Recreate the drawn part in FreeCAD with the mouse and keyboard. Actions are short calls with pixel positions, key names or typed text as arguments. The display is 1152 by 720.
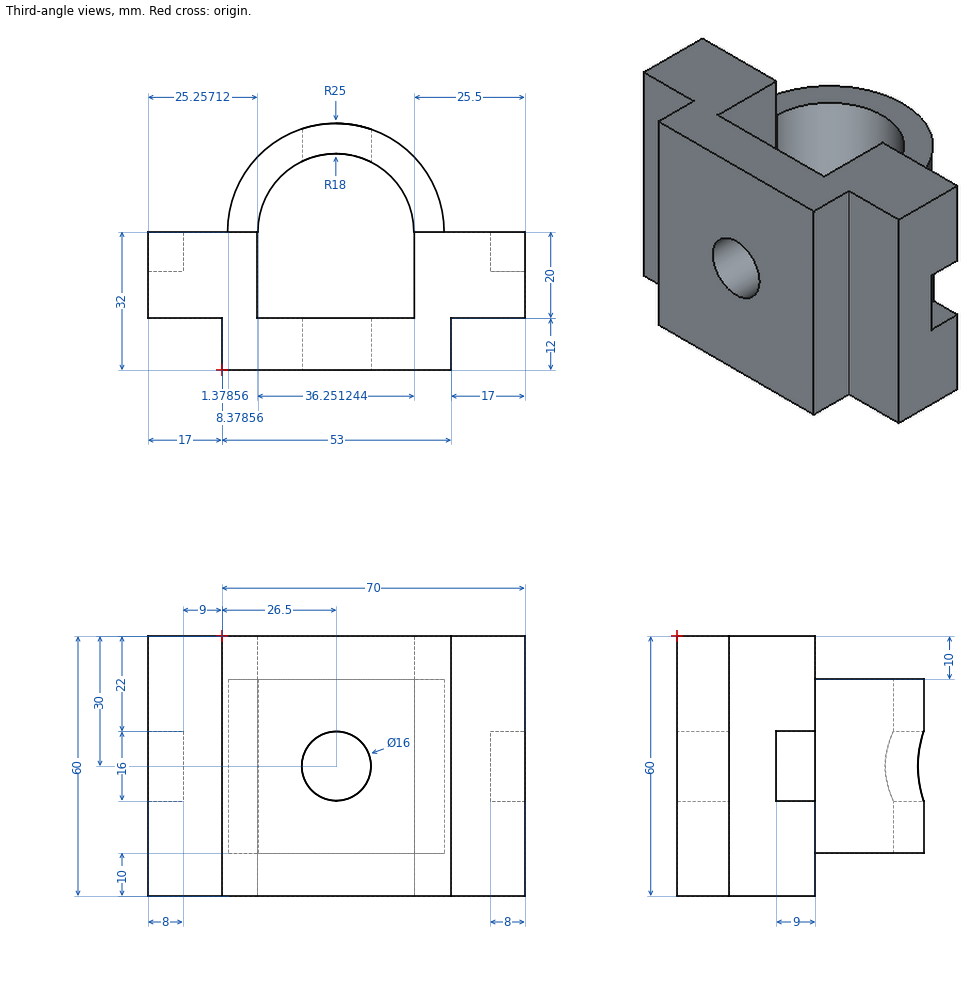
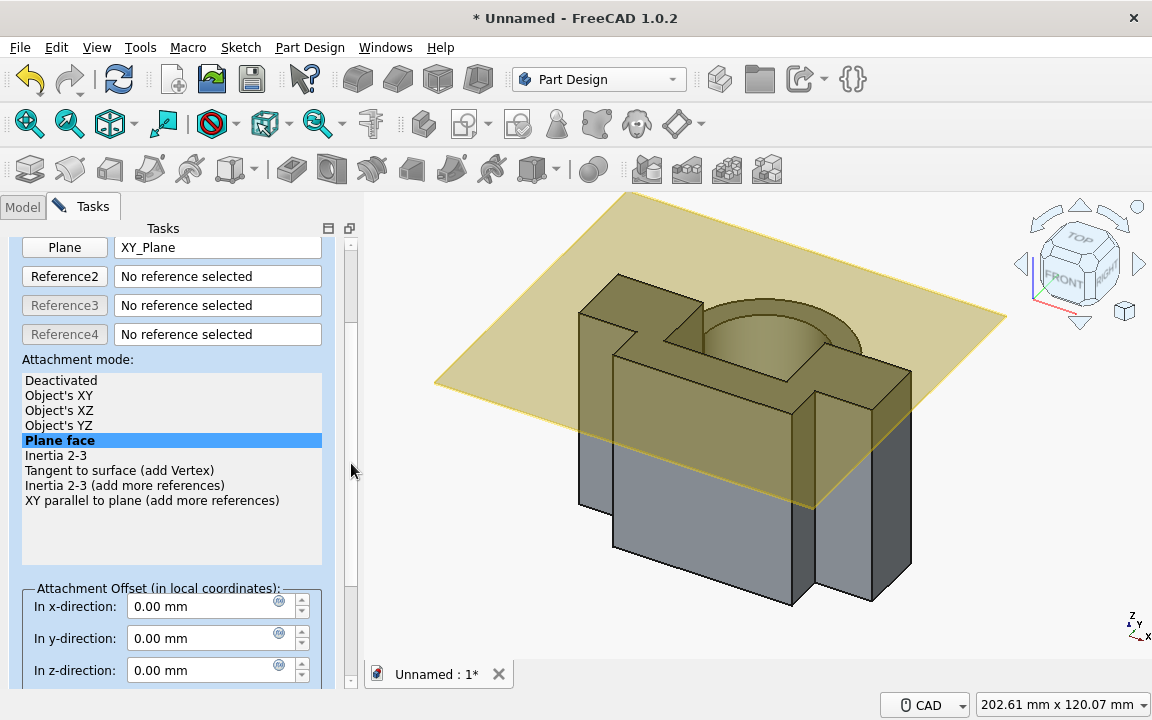
triple_click(210, 610)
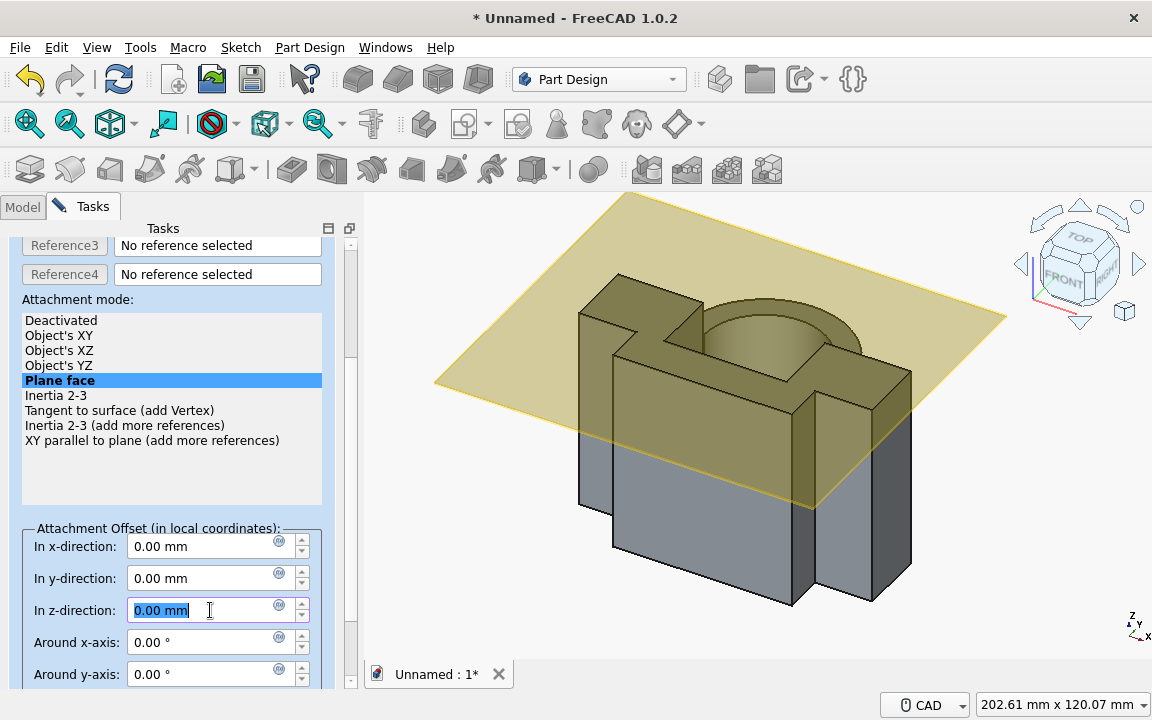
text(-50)
key(Tab)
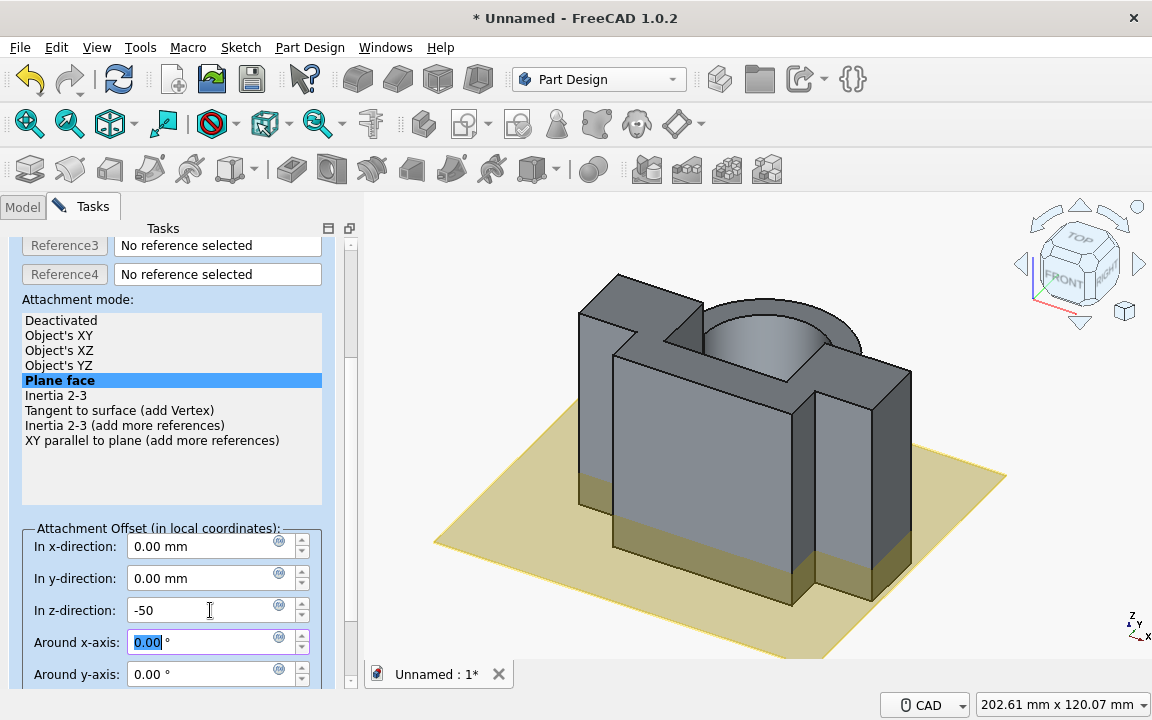
scroll(351, 463, up, 4)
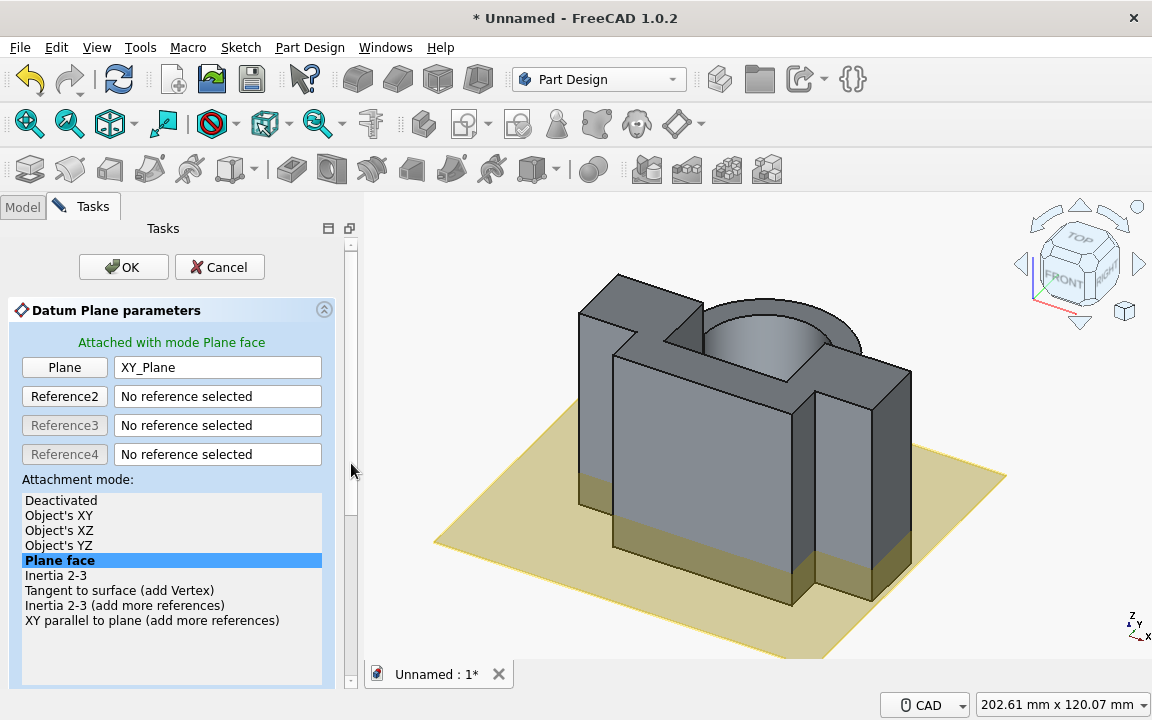
click(124, 267)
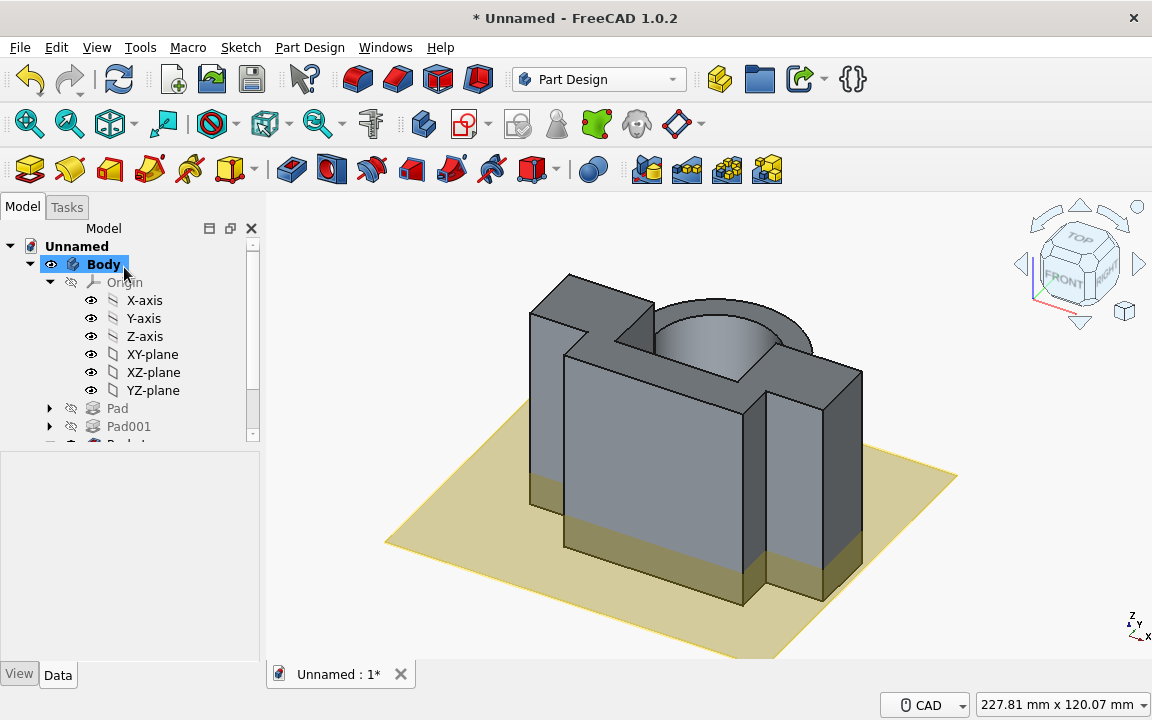
scroll(100, 332, down, 3)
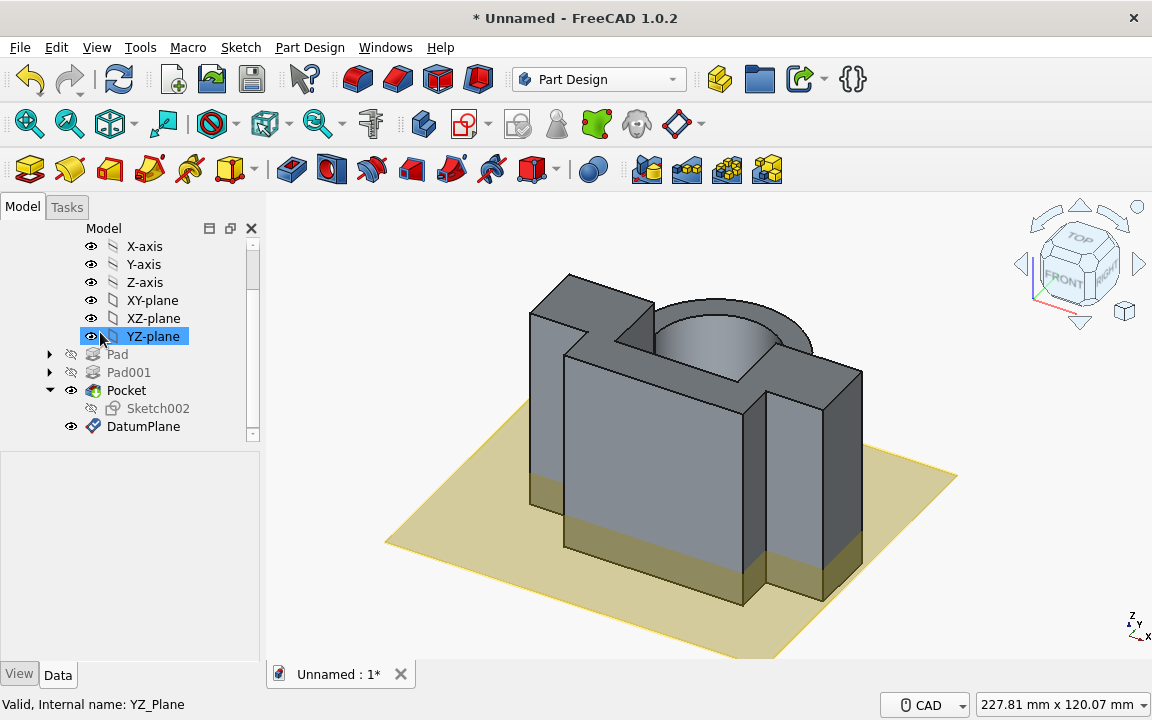
click(116, 426)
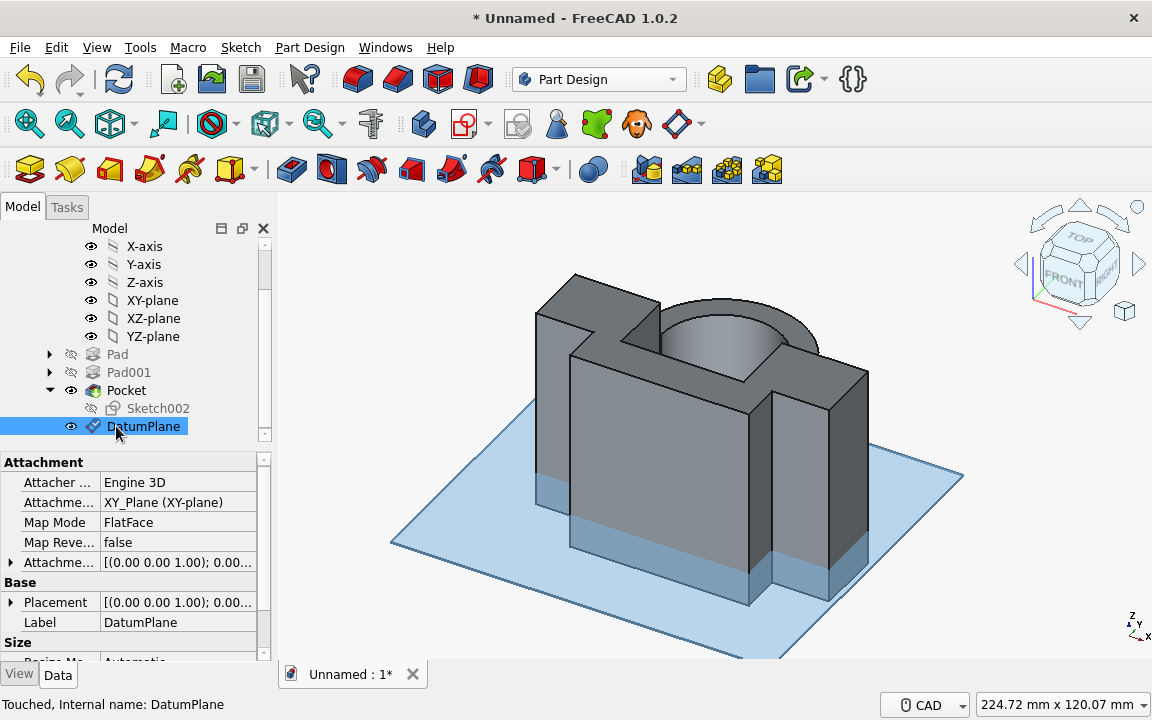
click(464, 124)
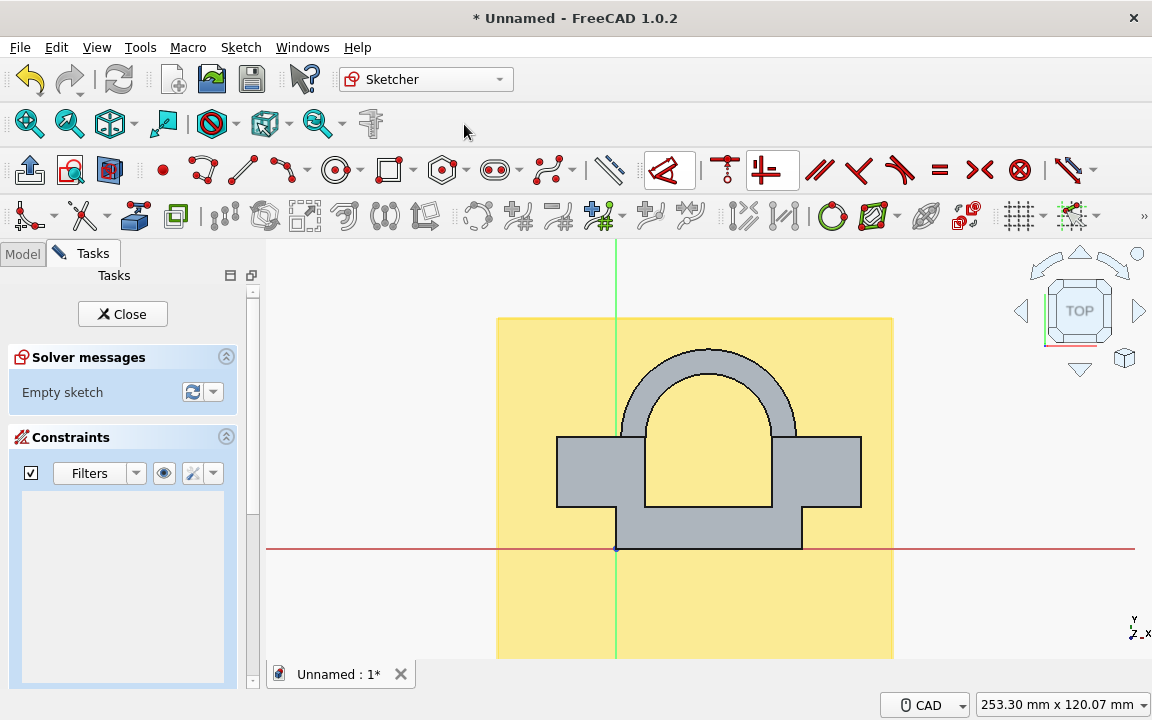
key(q)
key(s)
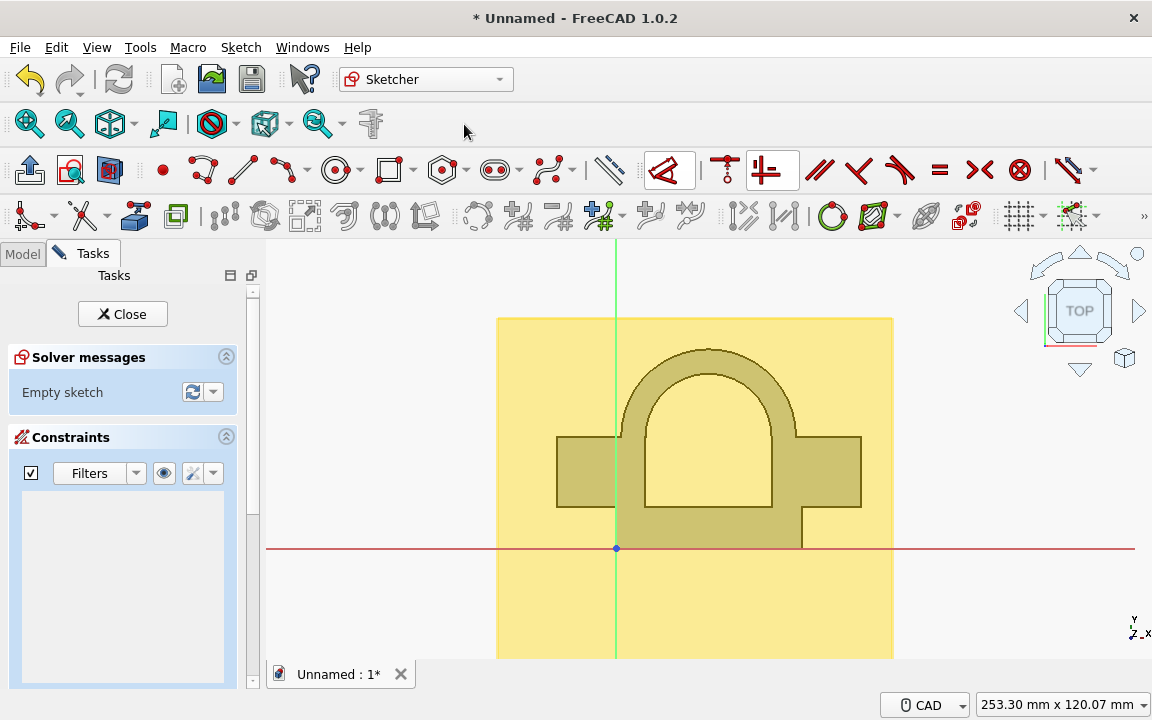
key(g)
key(l)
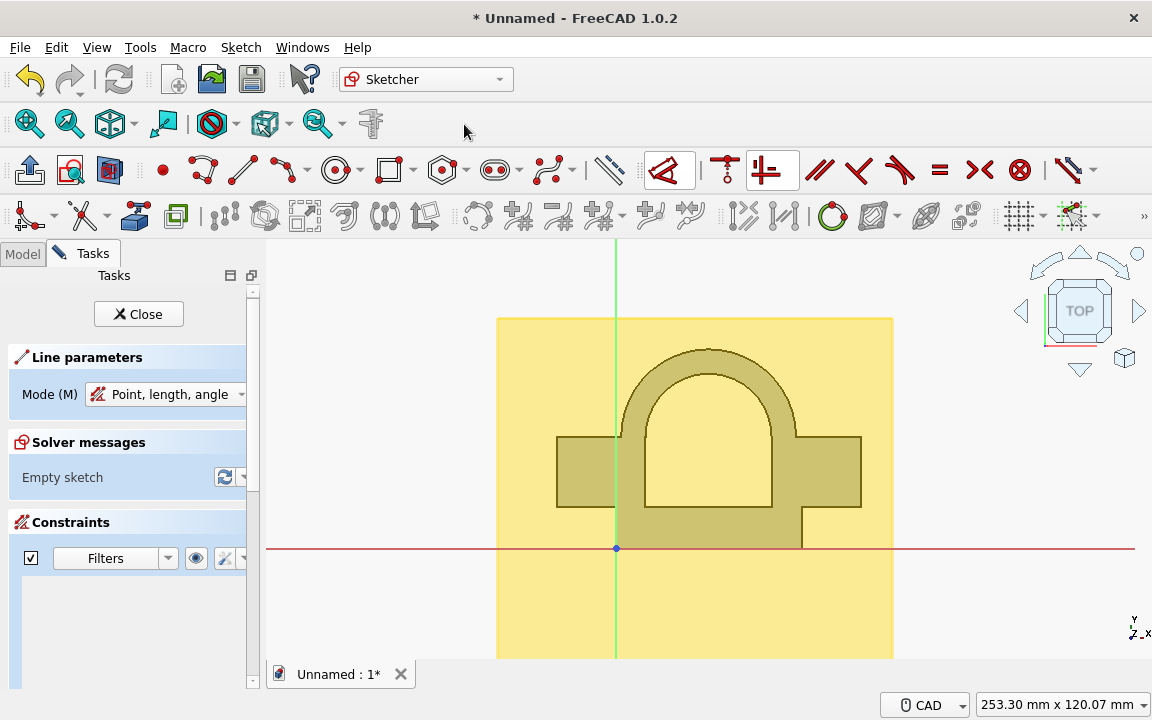
click(796, 437)
click(772, 437)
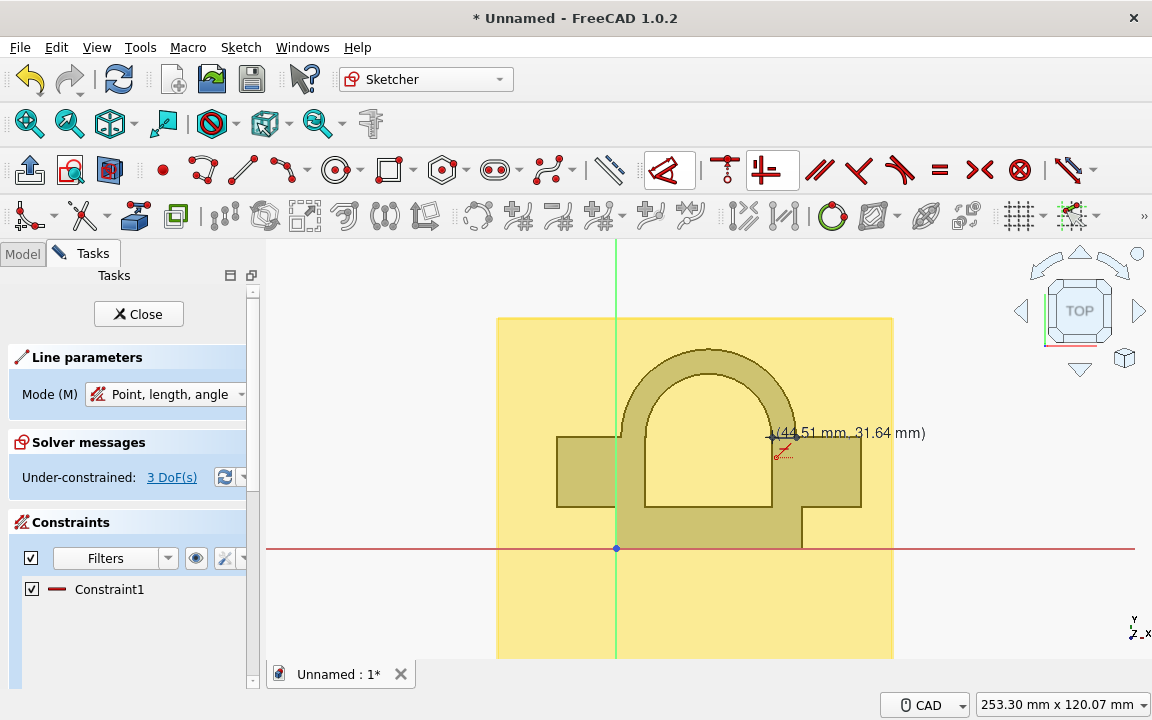
click(646, 437)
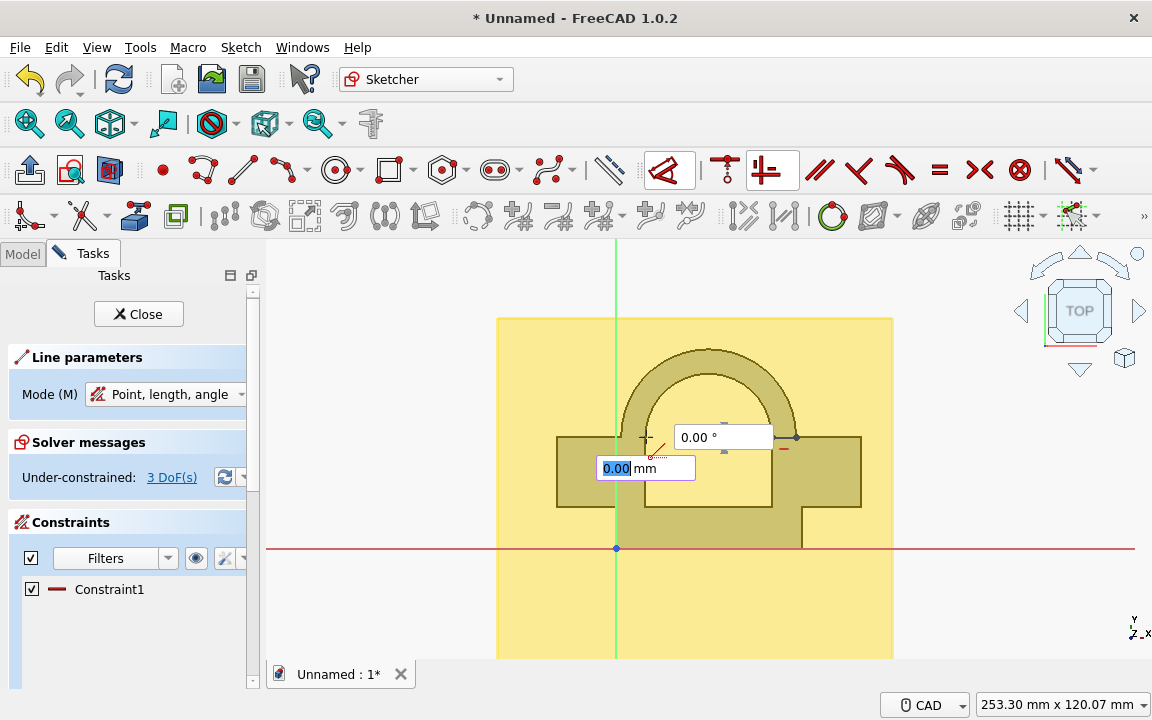
scroll(621, 437, up, 6)